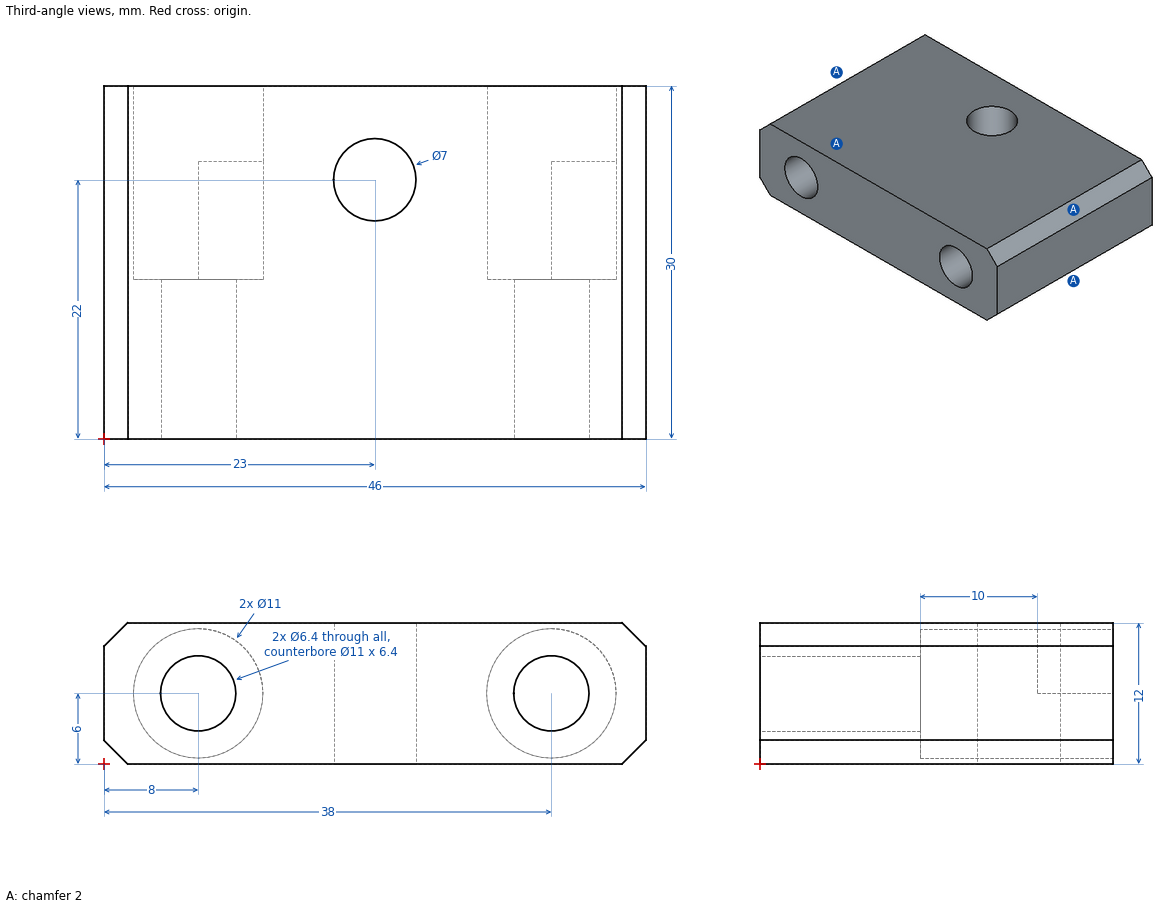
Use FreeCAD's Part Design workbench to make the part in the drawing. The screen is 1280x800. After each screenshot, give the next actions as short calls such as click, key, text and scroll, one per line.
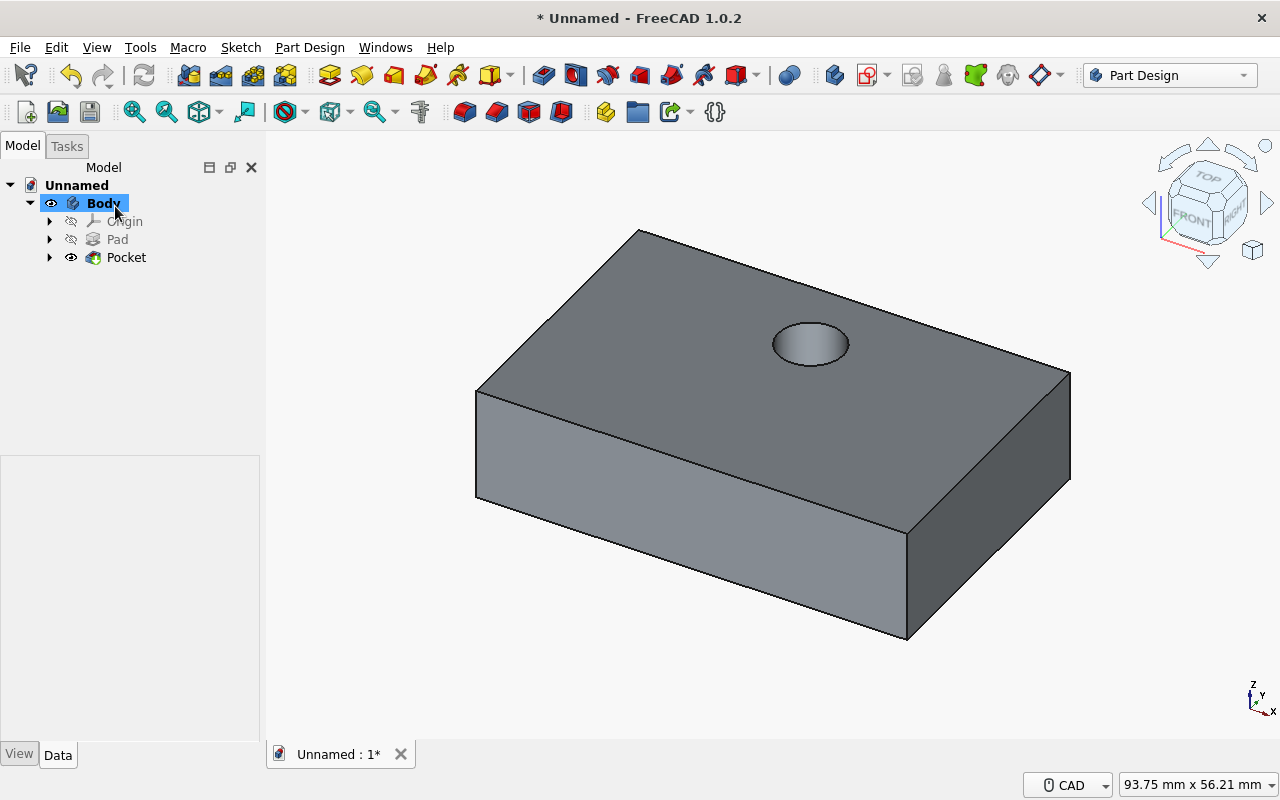
key(4)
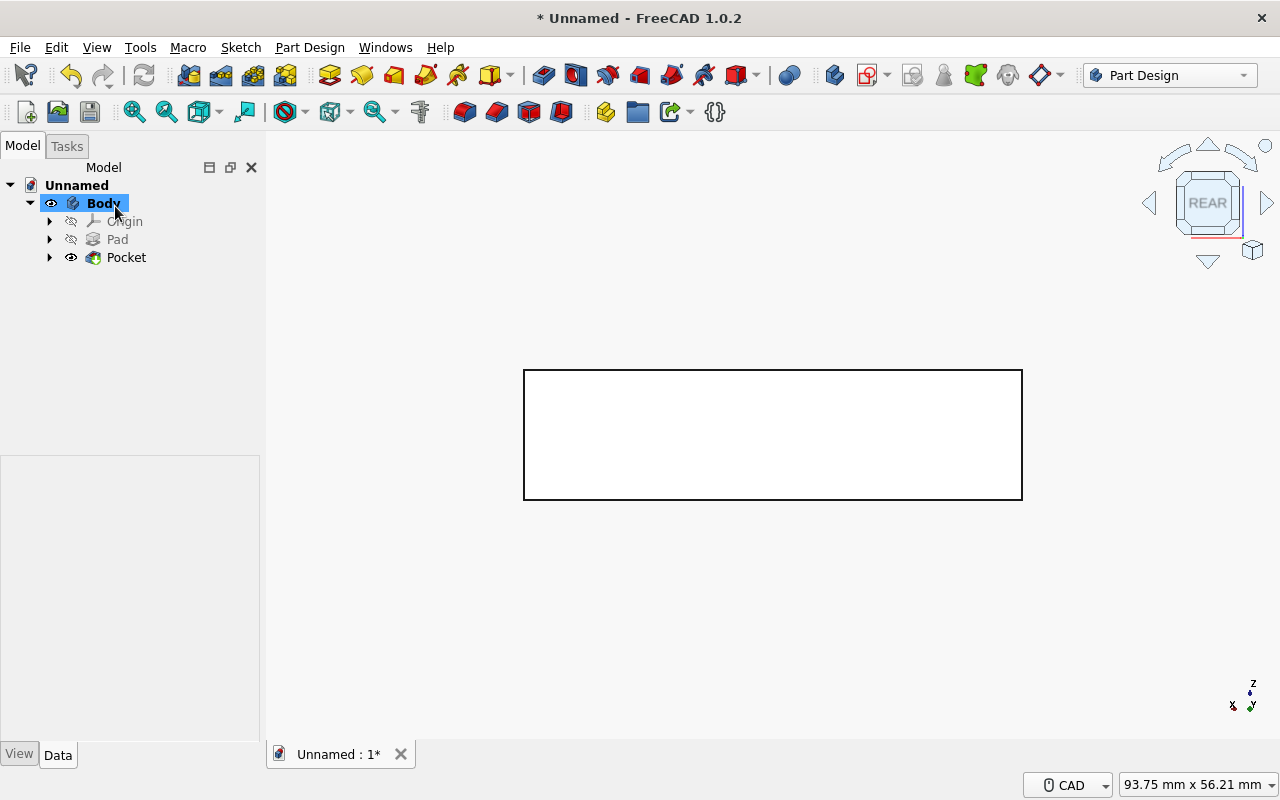
click(631, 434)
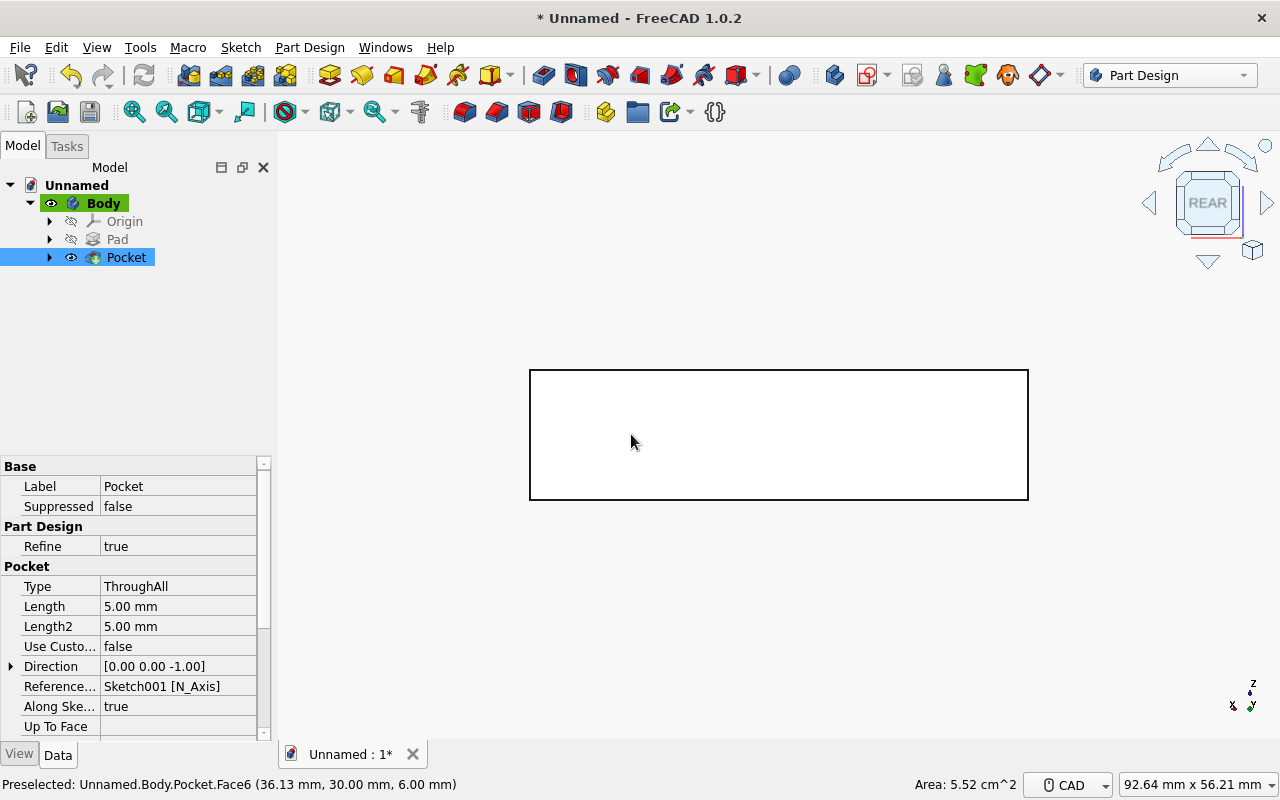
click(868, 76)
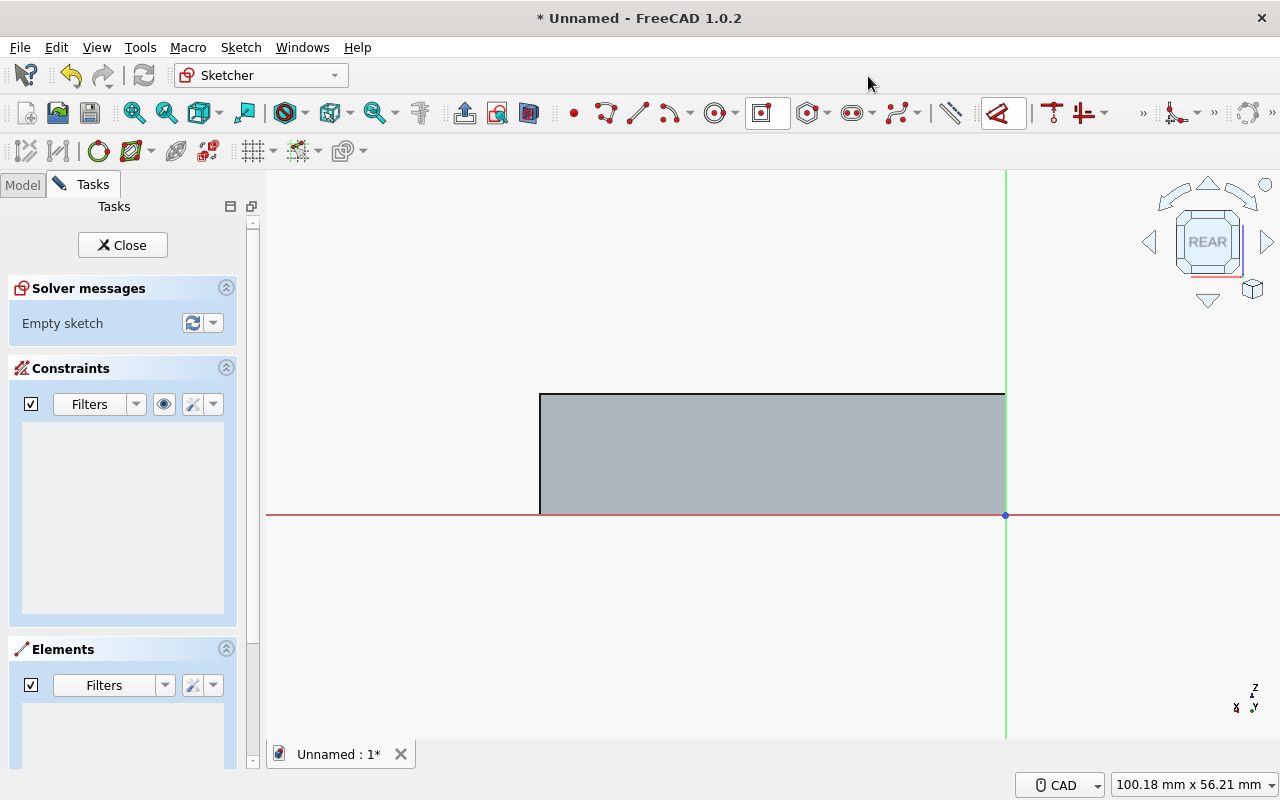
scroll(986, 497, up, 2)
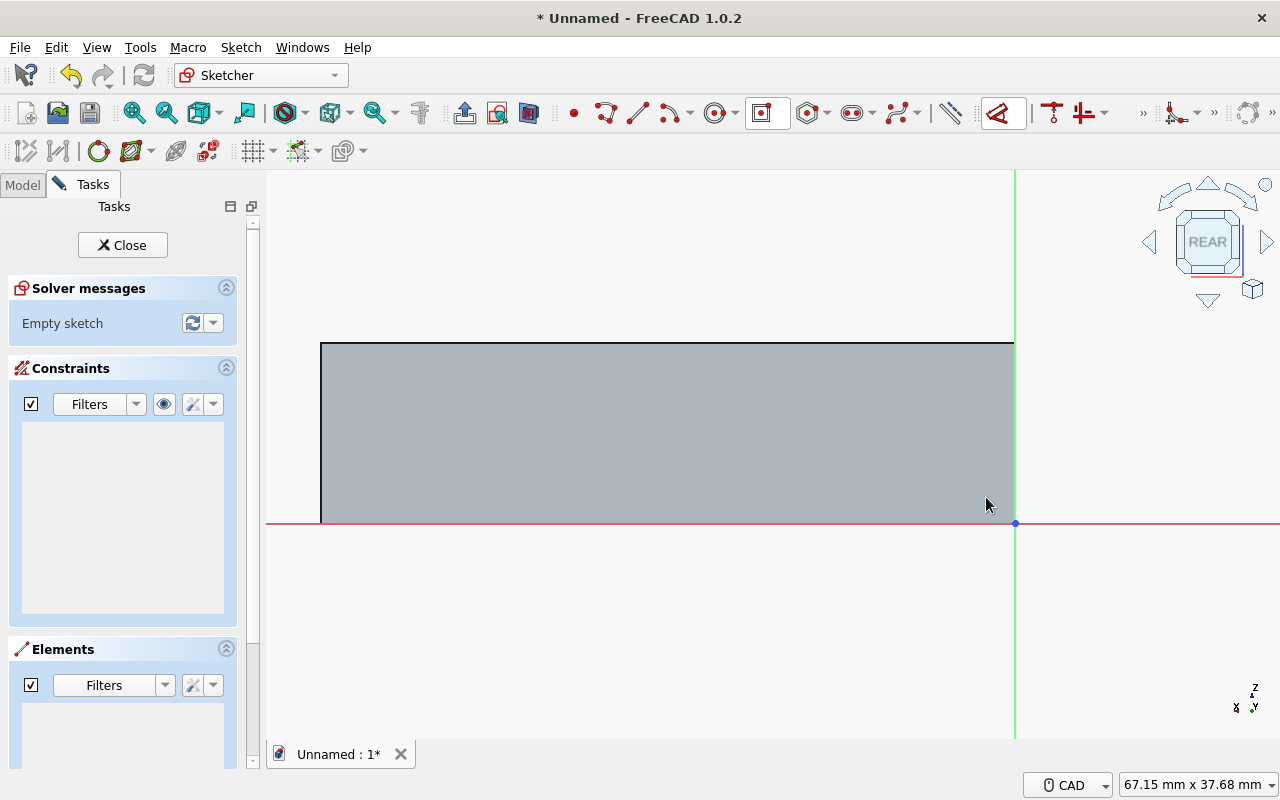
key(g)
key(c)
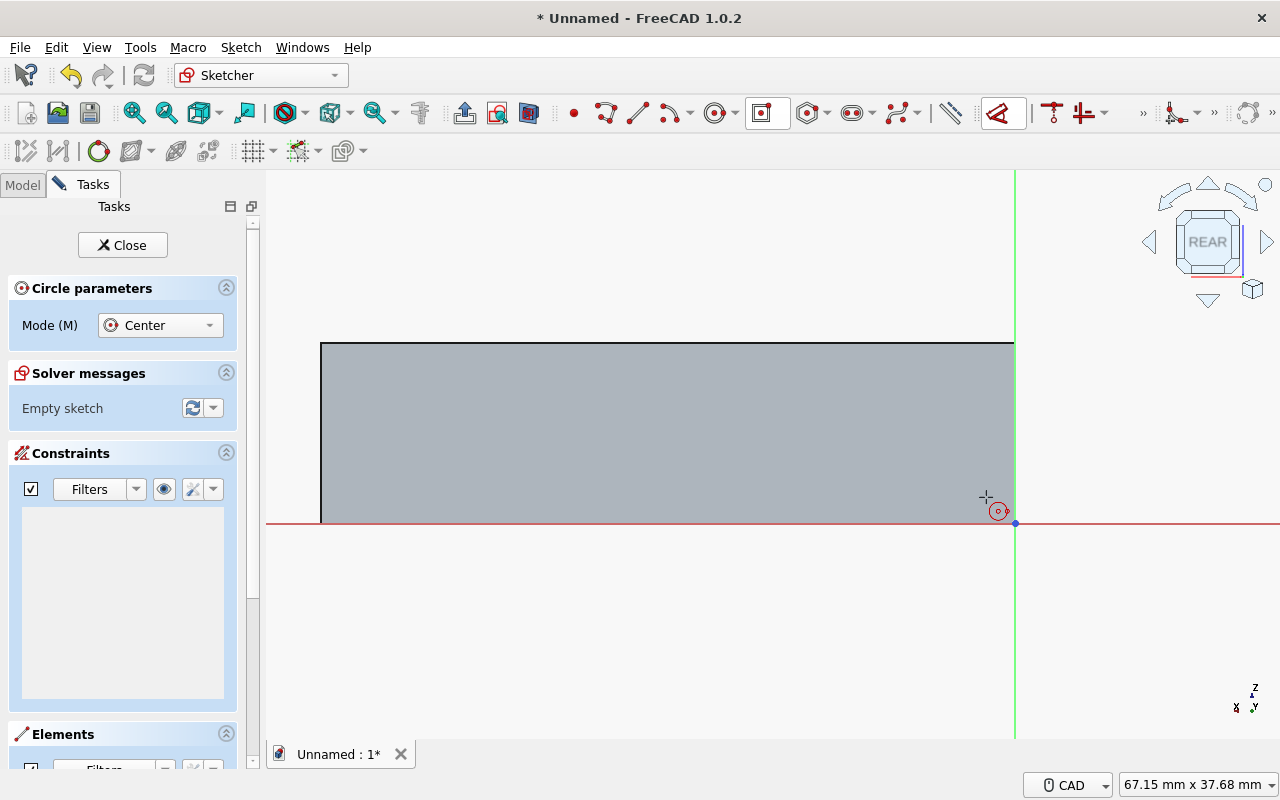
click(894, 433)
move(929, 399)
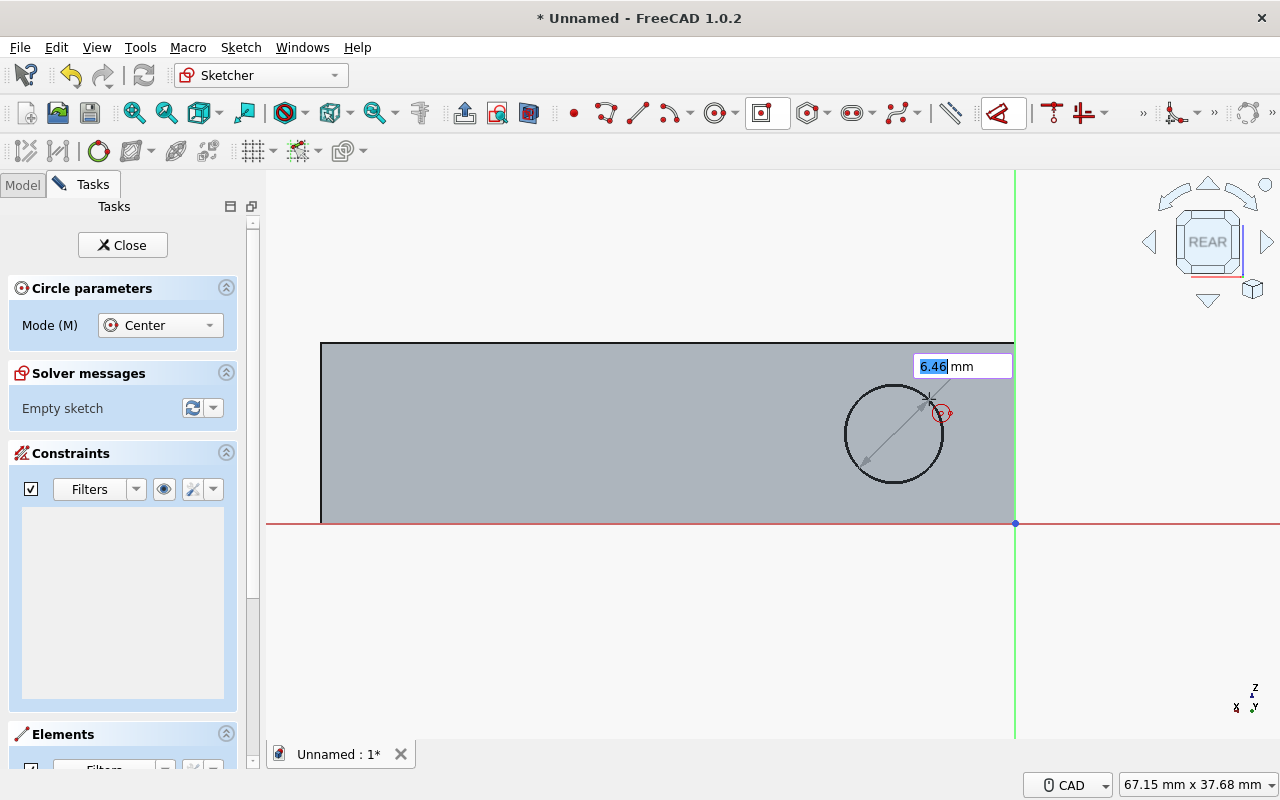
text(6.4)
key(Return)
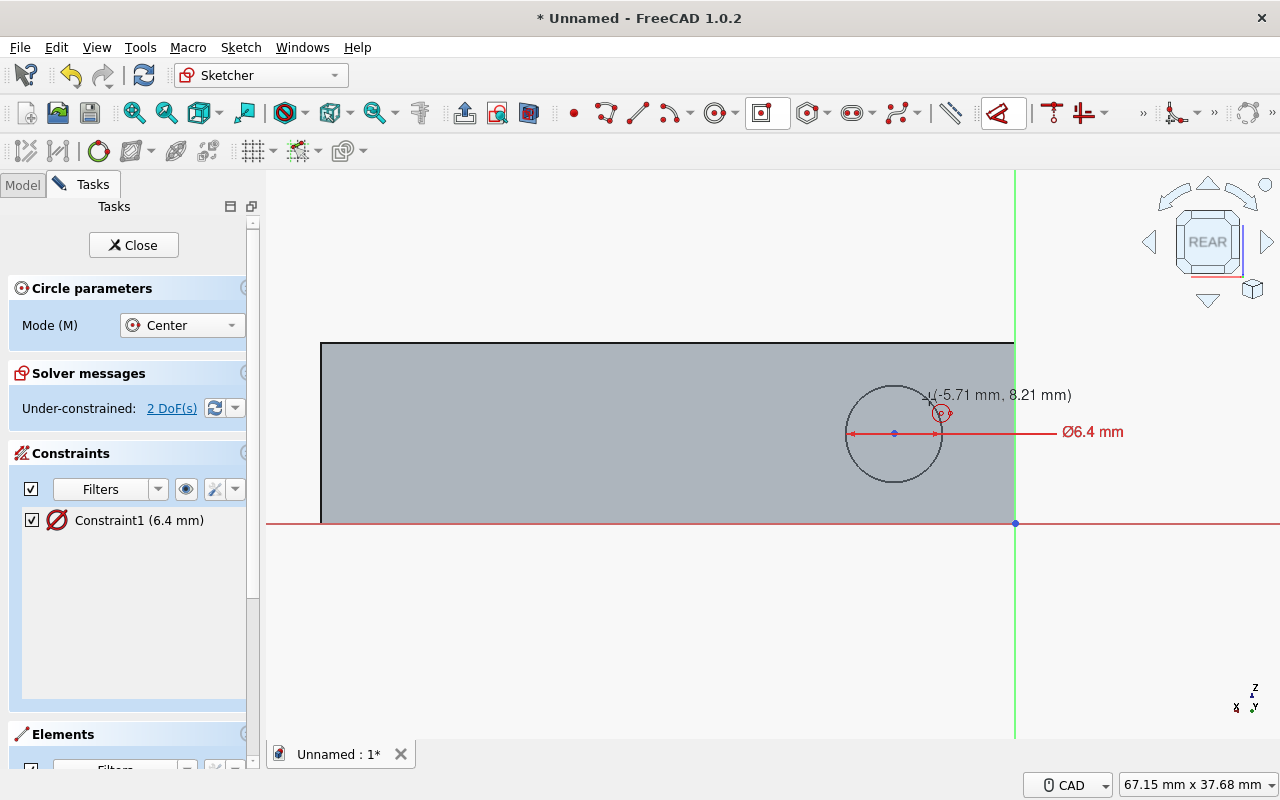
click(441, 433)
move(476, 399)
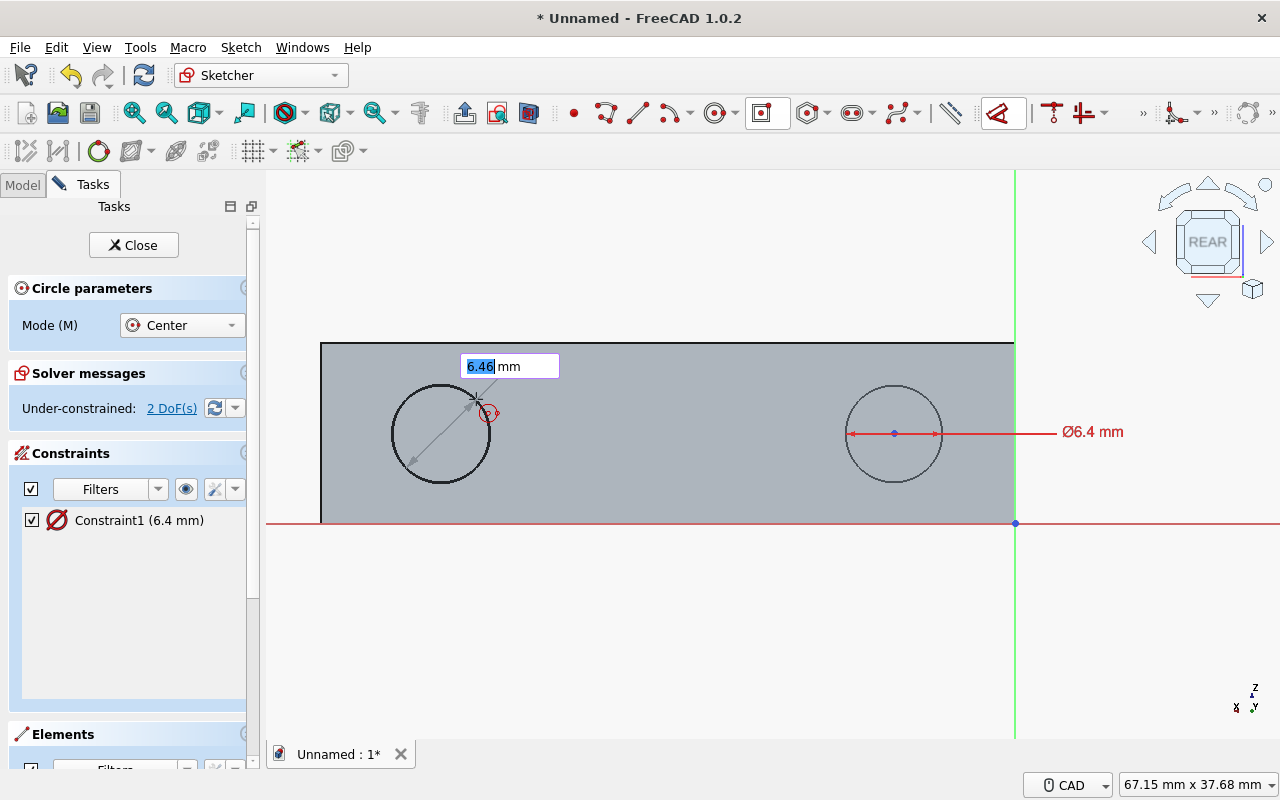
text(6.4)
key(Return)
key(Escape)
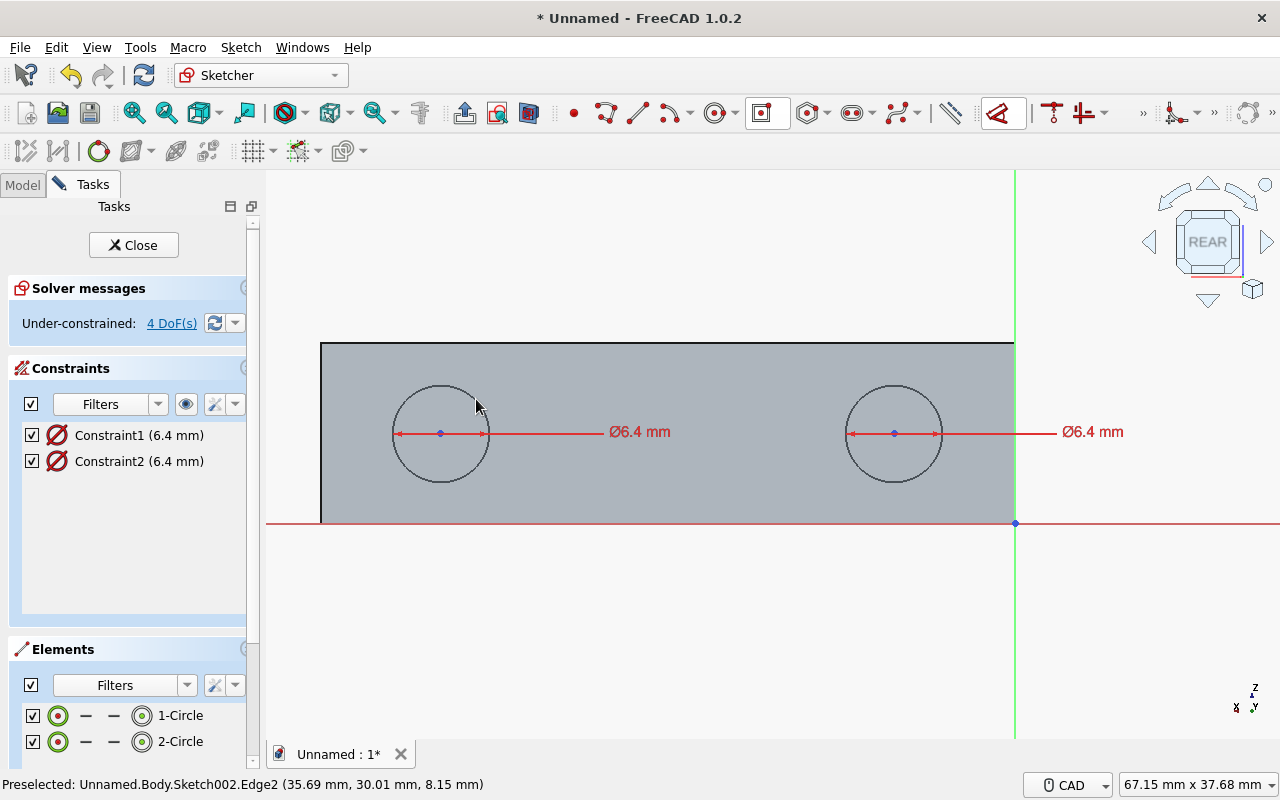
click(894, 434)